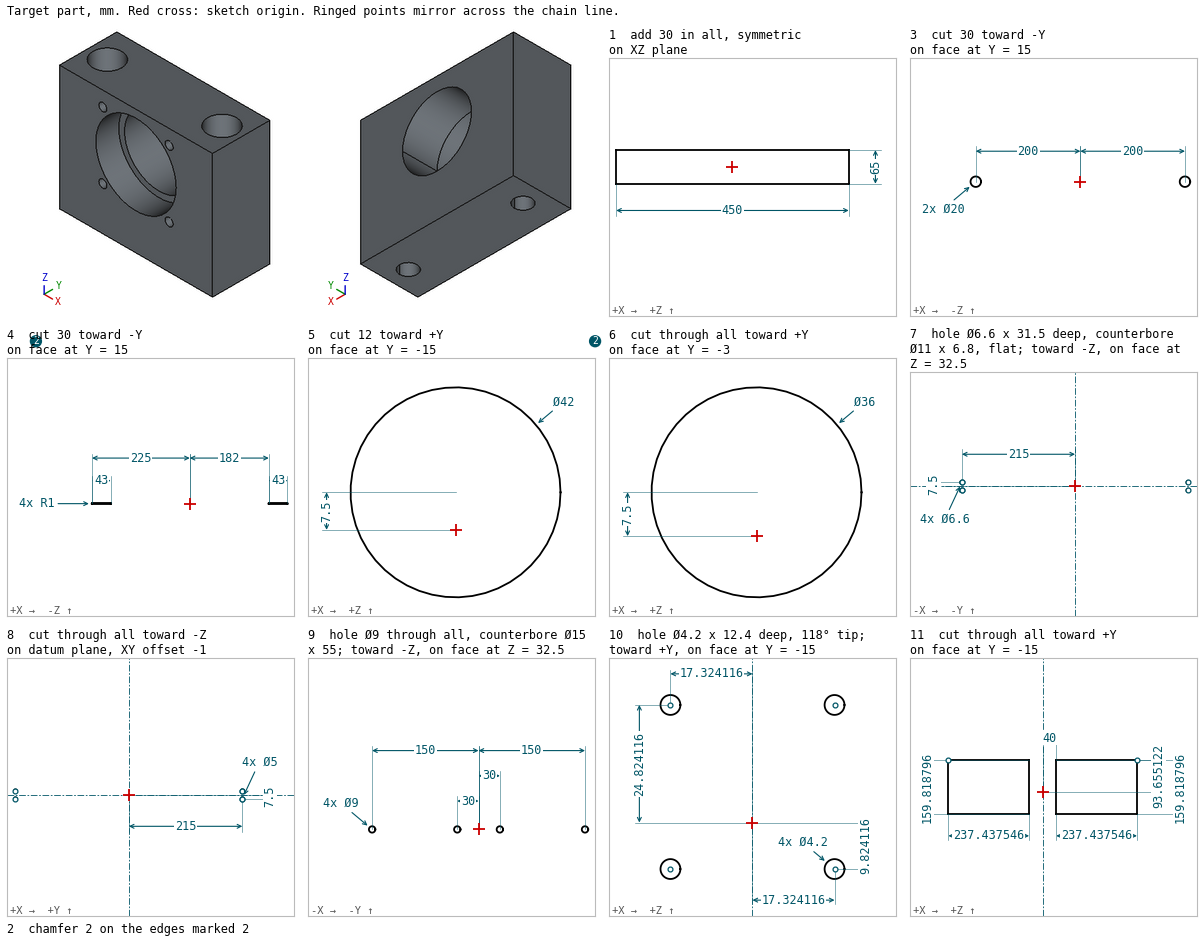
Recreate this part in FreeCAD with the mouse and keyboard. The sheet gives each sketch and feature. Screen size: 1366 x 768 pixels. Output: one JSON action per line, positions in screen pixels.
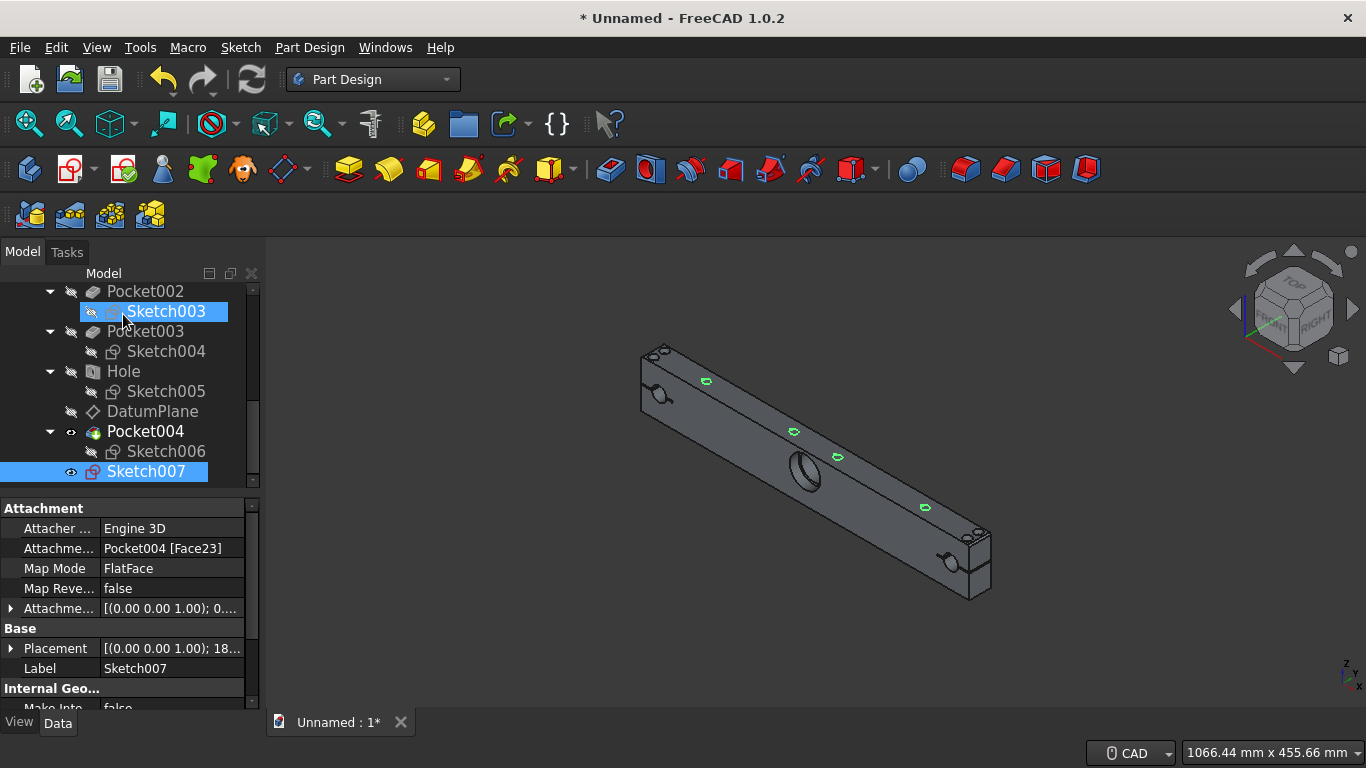
{"action": "left_click", "coordinate": [652, 170]}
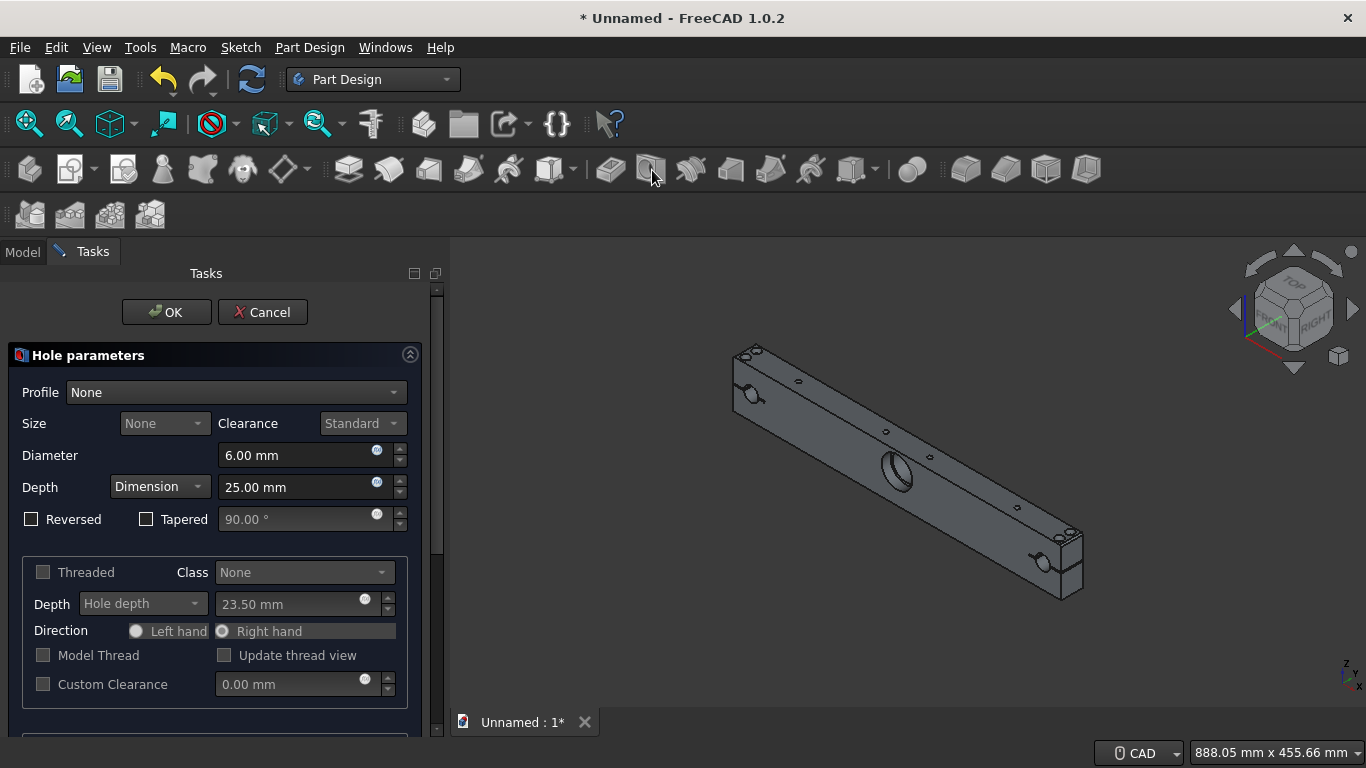
{"action": "triple_click", "coordinate": [305, 455]}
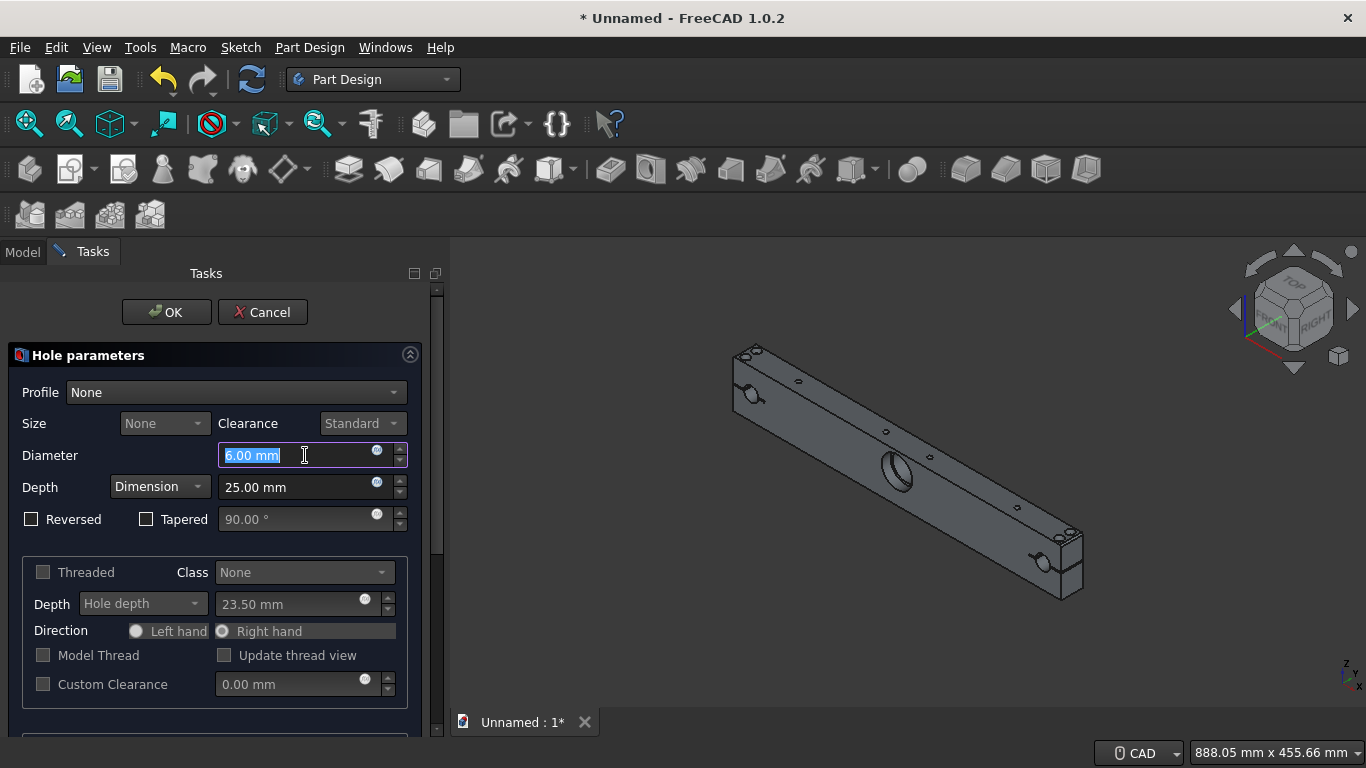
{"action": "type", "text": "9"}
{"action": "key", "text": "Tab"}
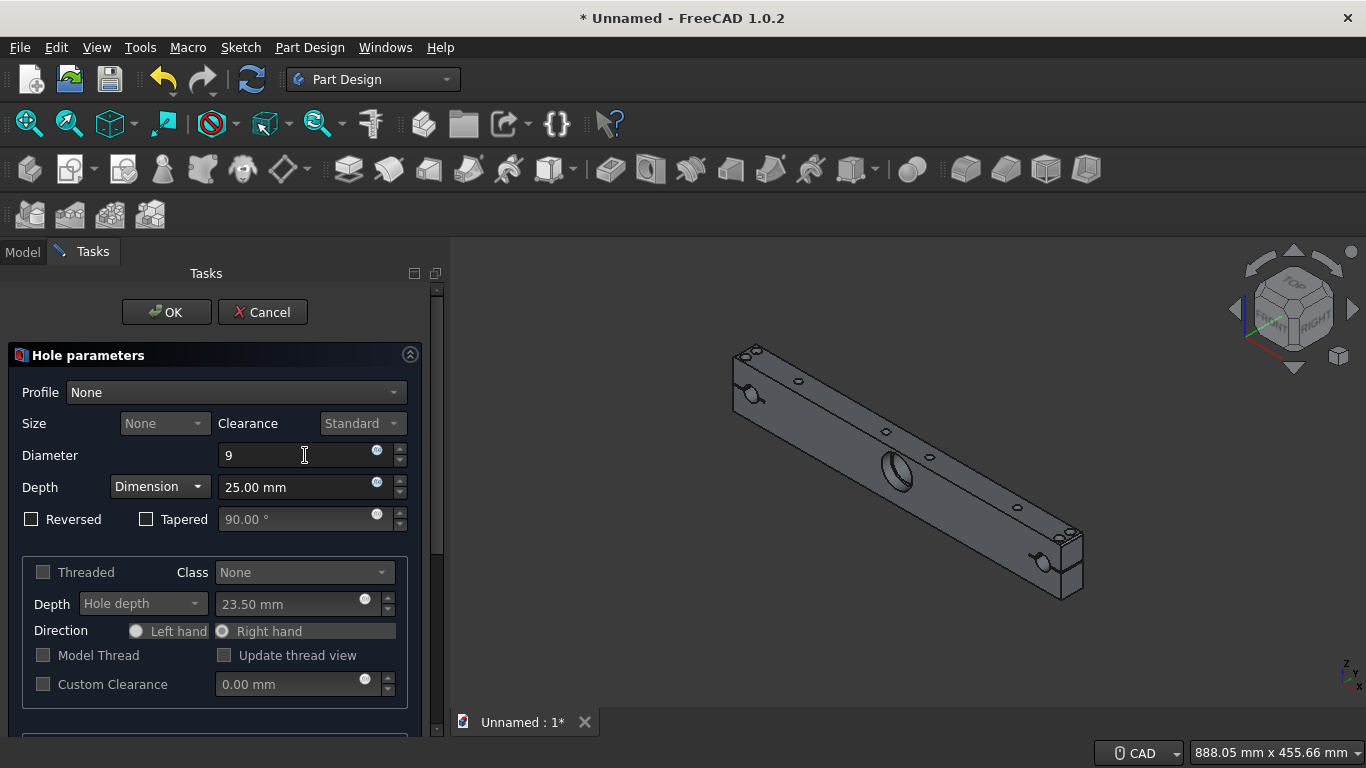
{"action": "left_click", "coordinate": [161, 486]}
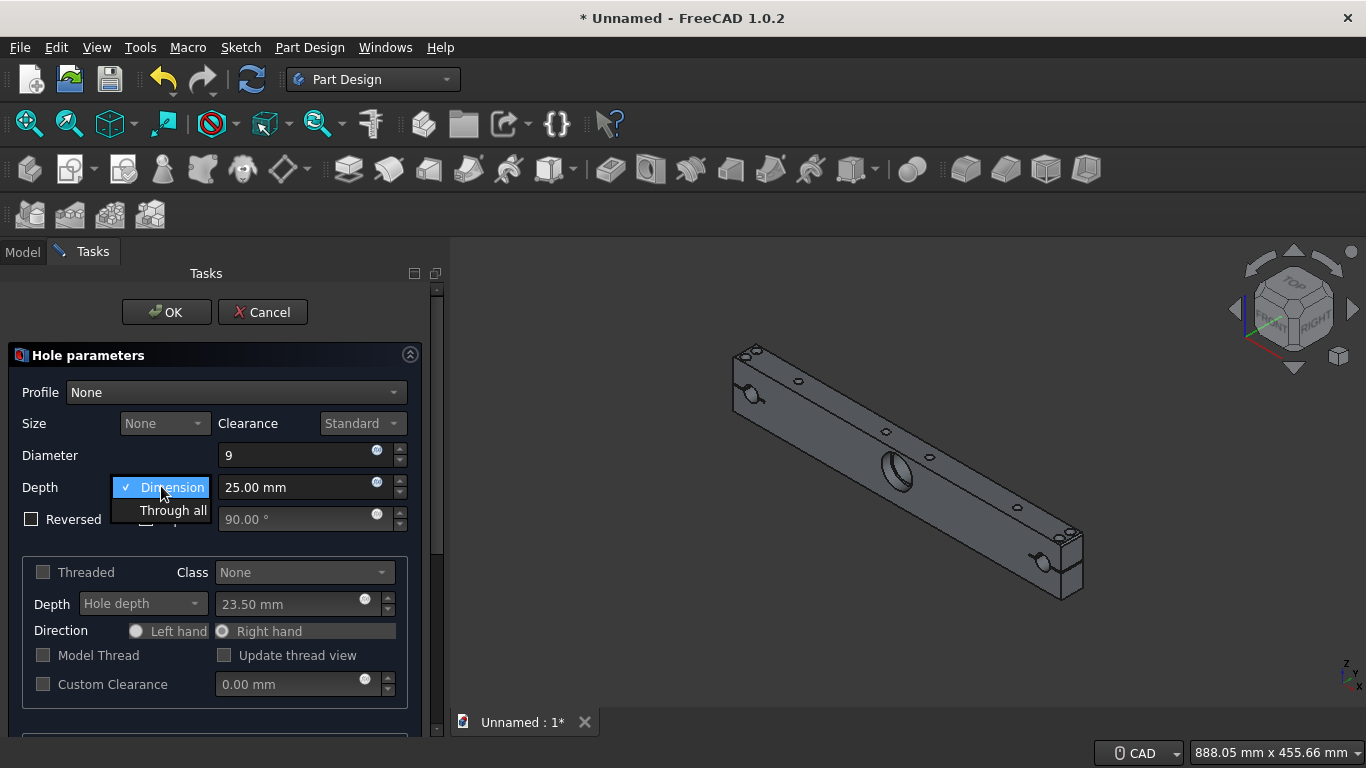
{"action": "left_click", "coordinate": [160, 510]}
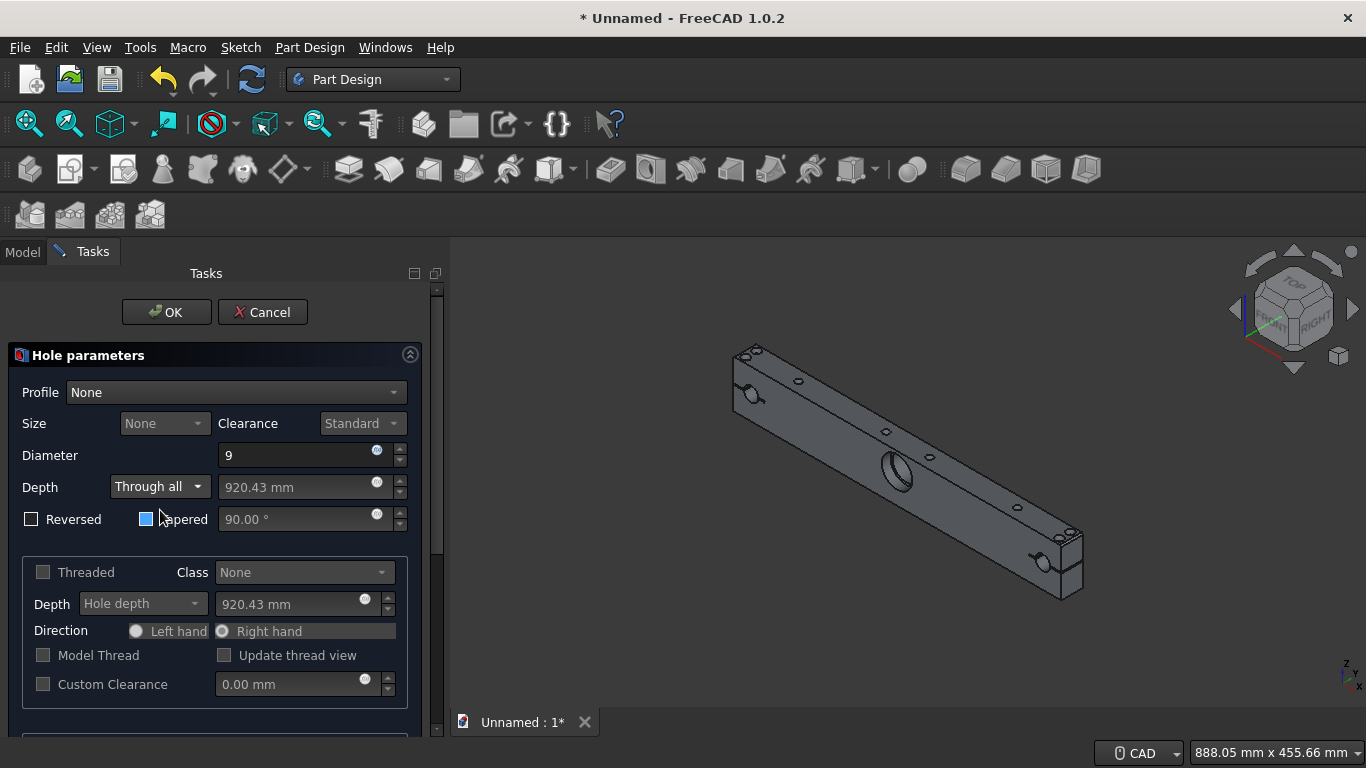
{"action": "scroll", "coordinate": [437, 510], "scroll_direction": "down", "scroll_amount": 2}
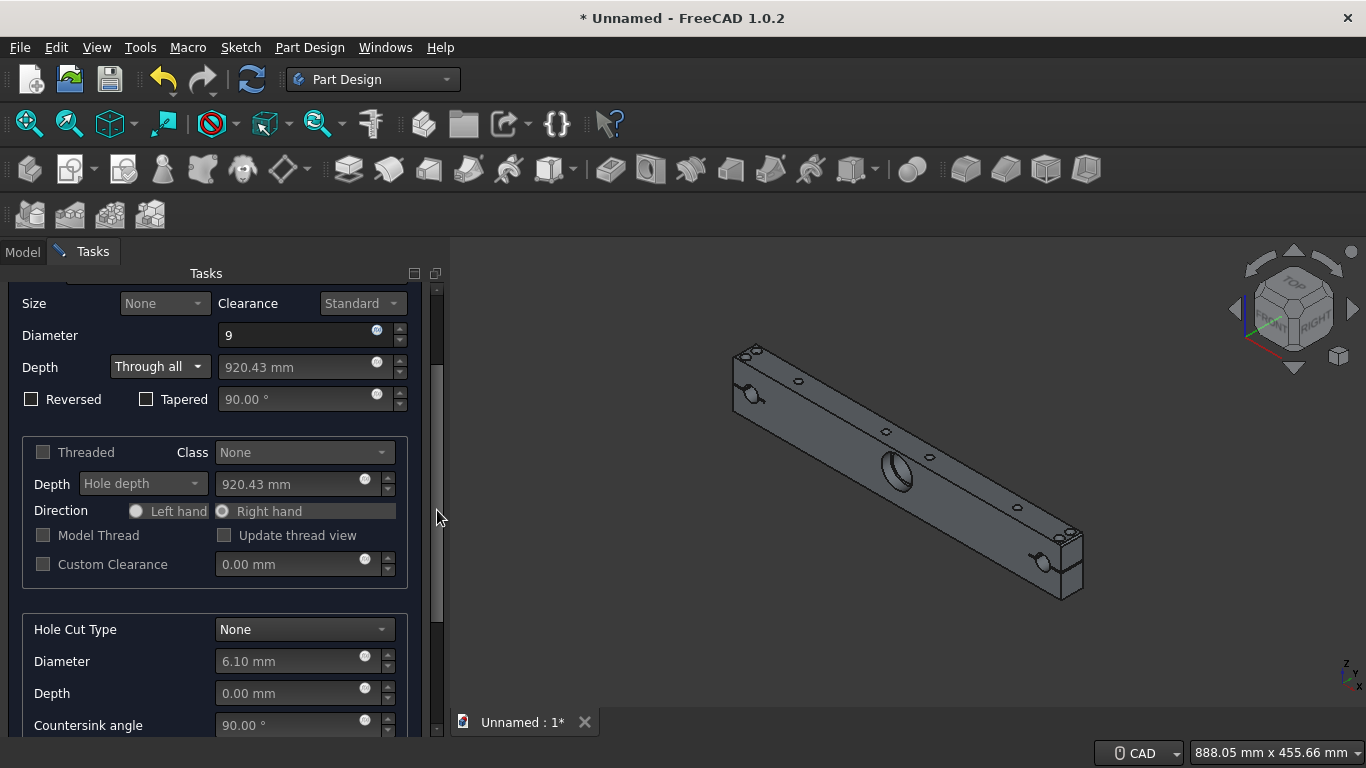
{"action": "left_click", "coordinate": [306, 630]}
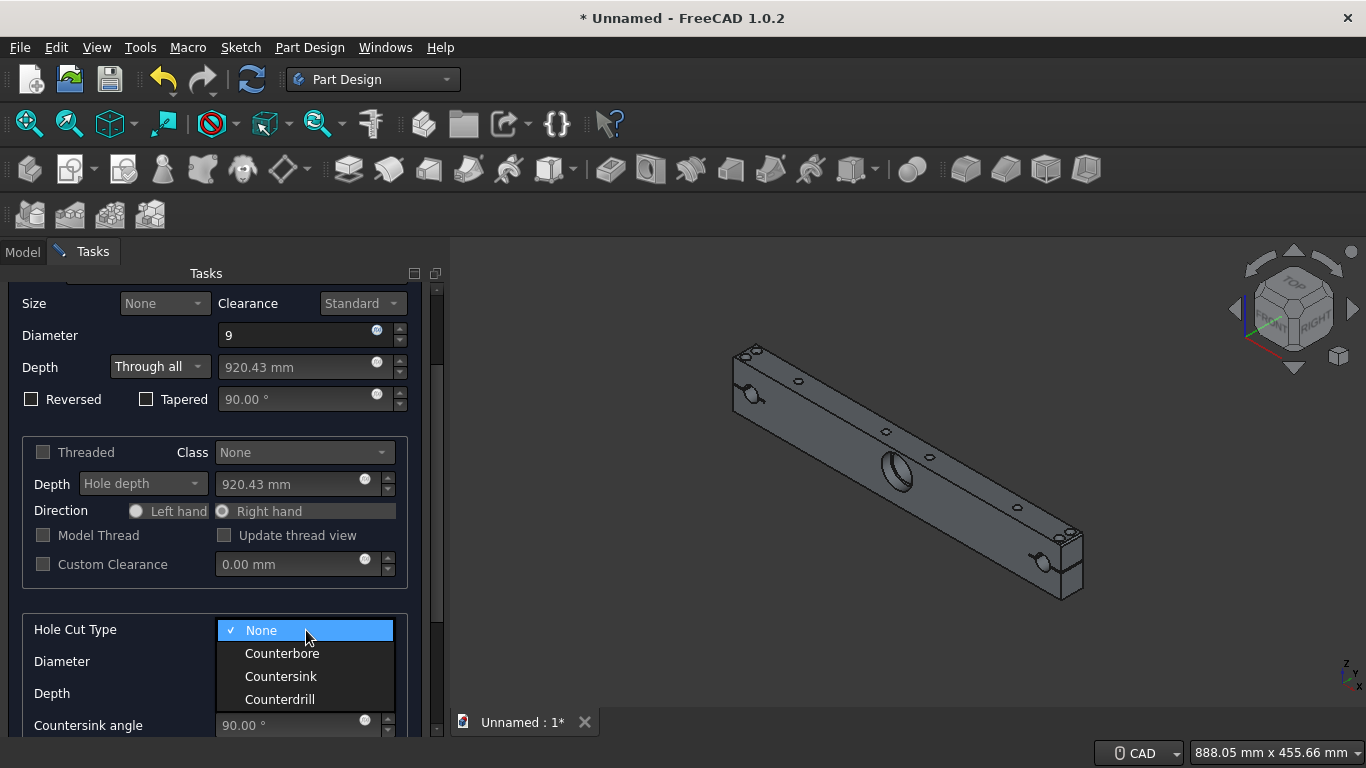
{"action": "left_click", "coordinate": [304, 654]}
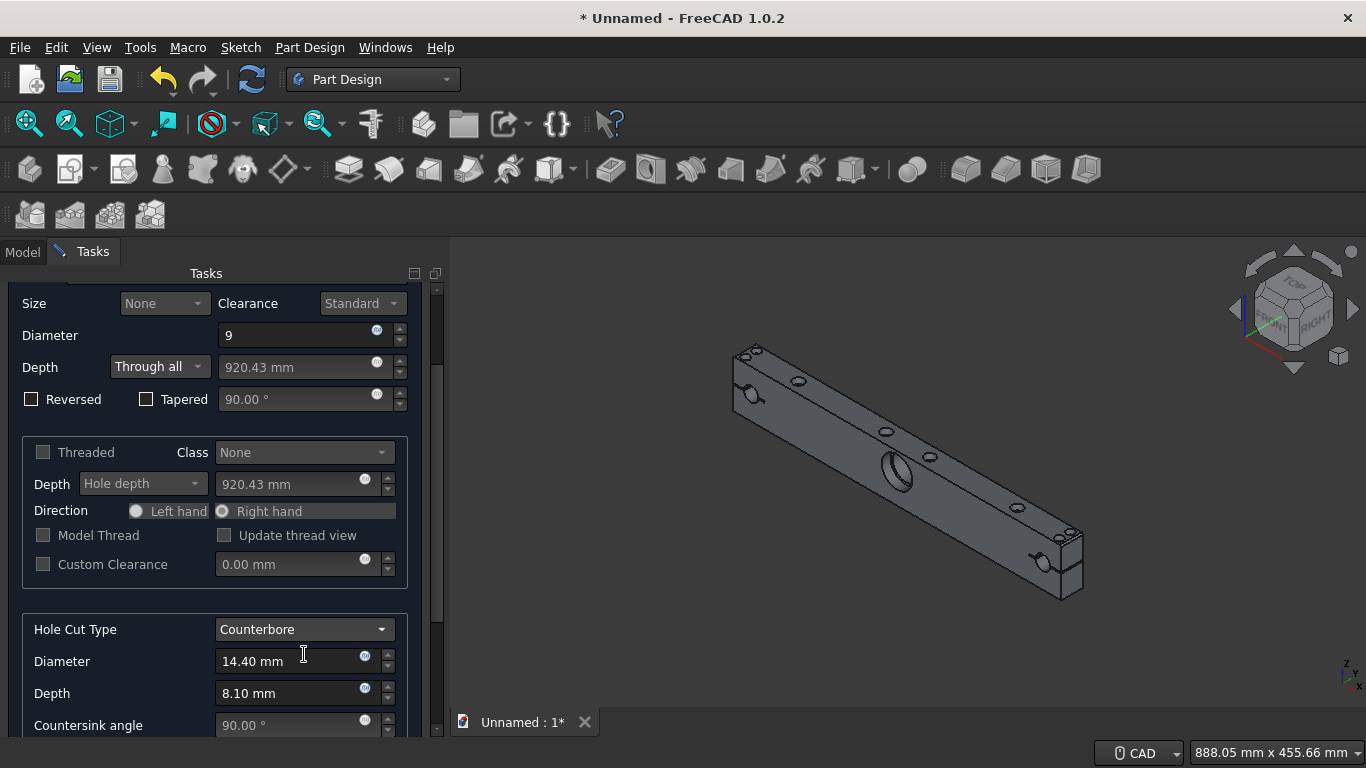
{"action": "triple_click", "coordinate": [298, 661]}